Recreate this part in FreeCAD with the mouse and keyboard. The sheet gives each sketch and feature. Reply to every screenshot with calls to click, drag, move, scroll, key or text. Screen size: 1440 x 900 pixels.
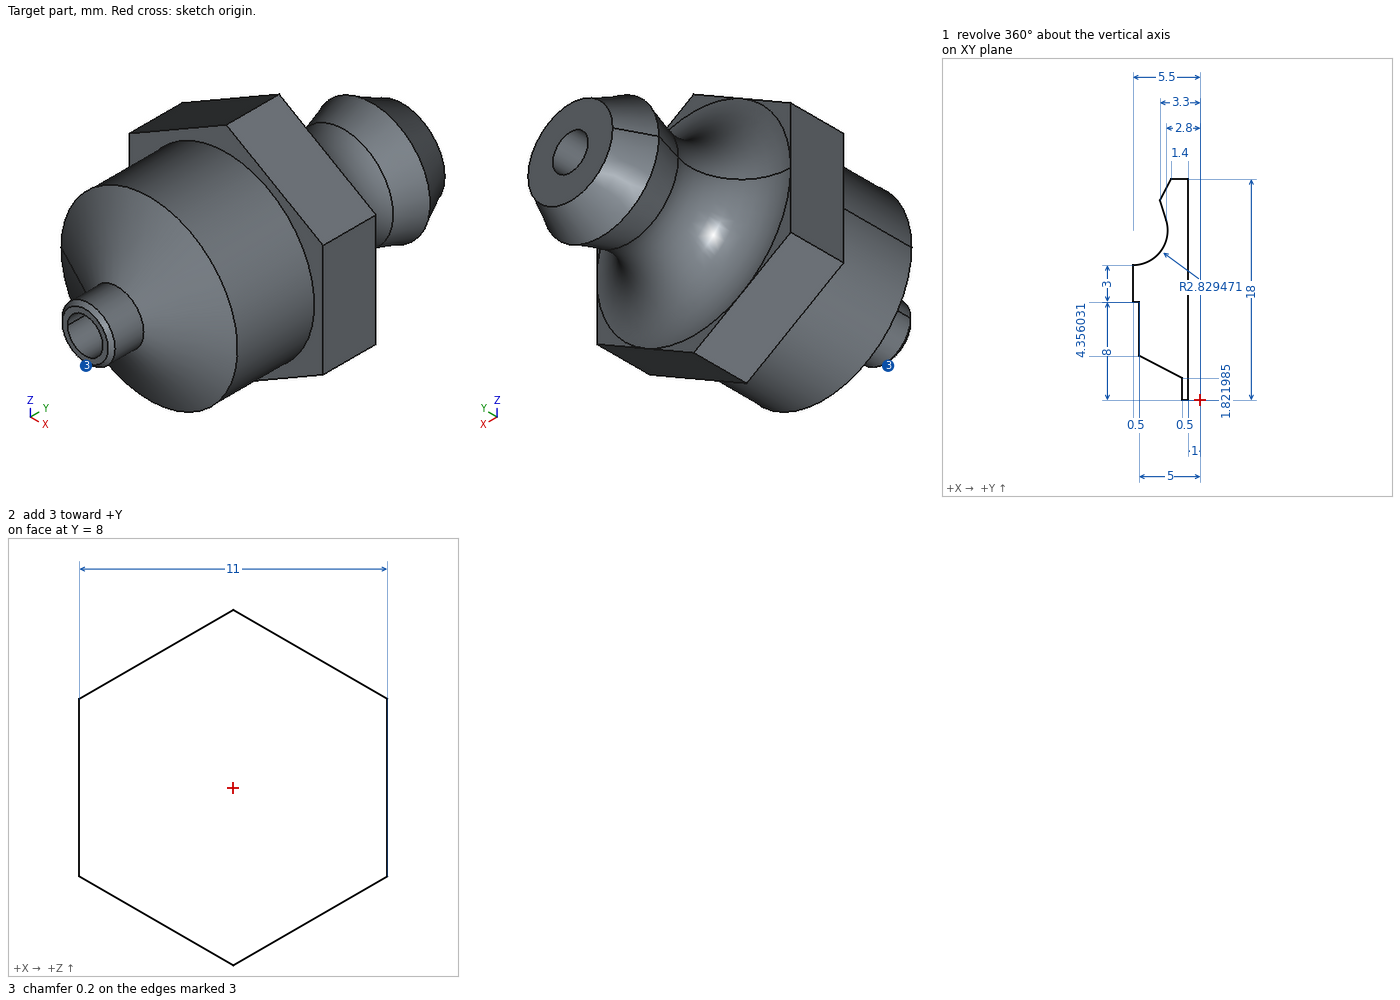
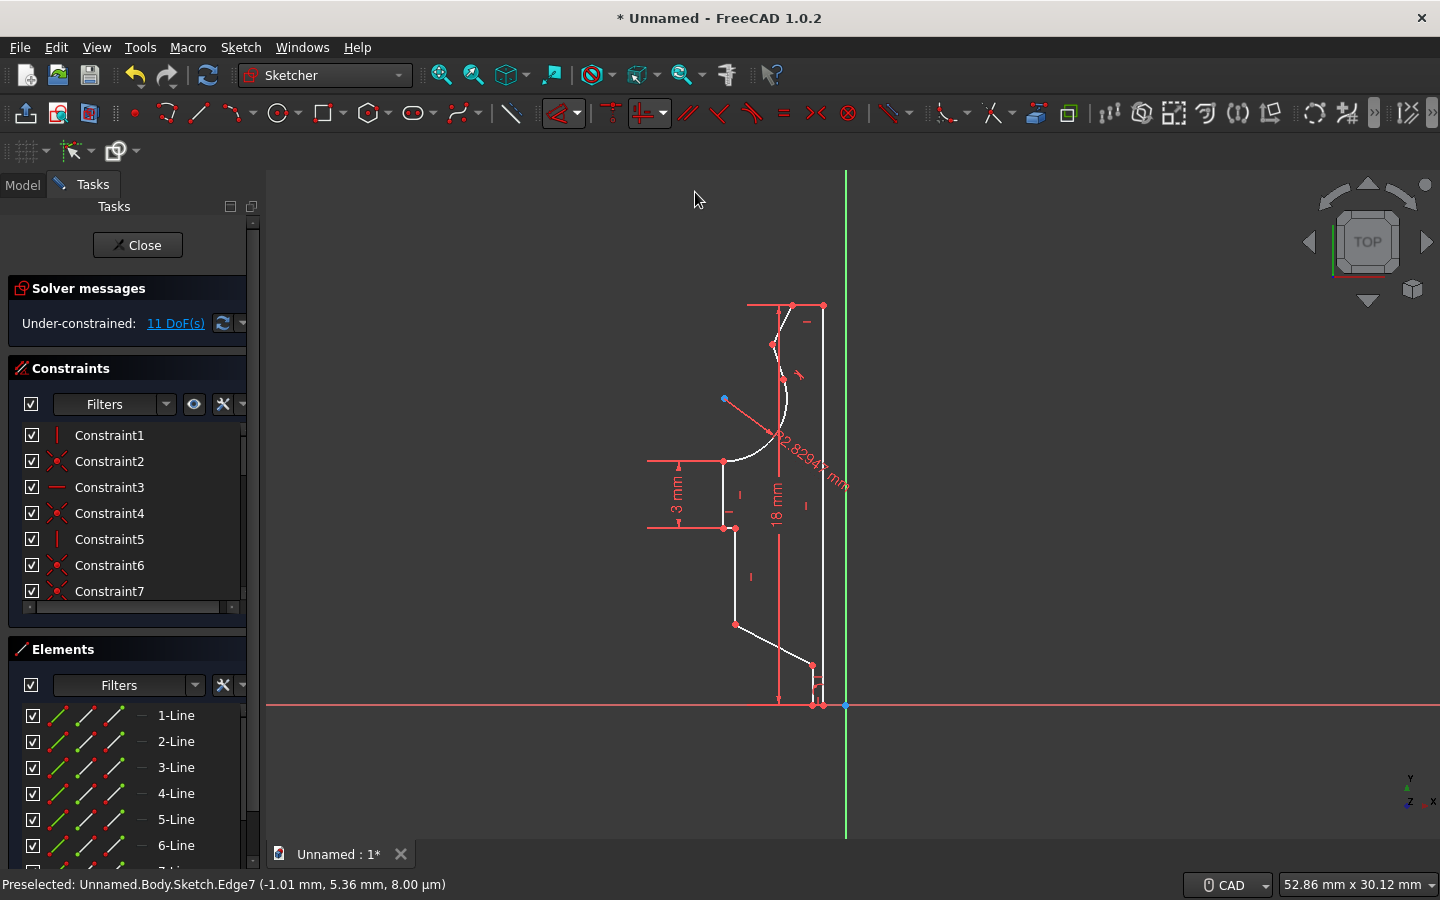
click(723, 528)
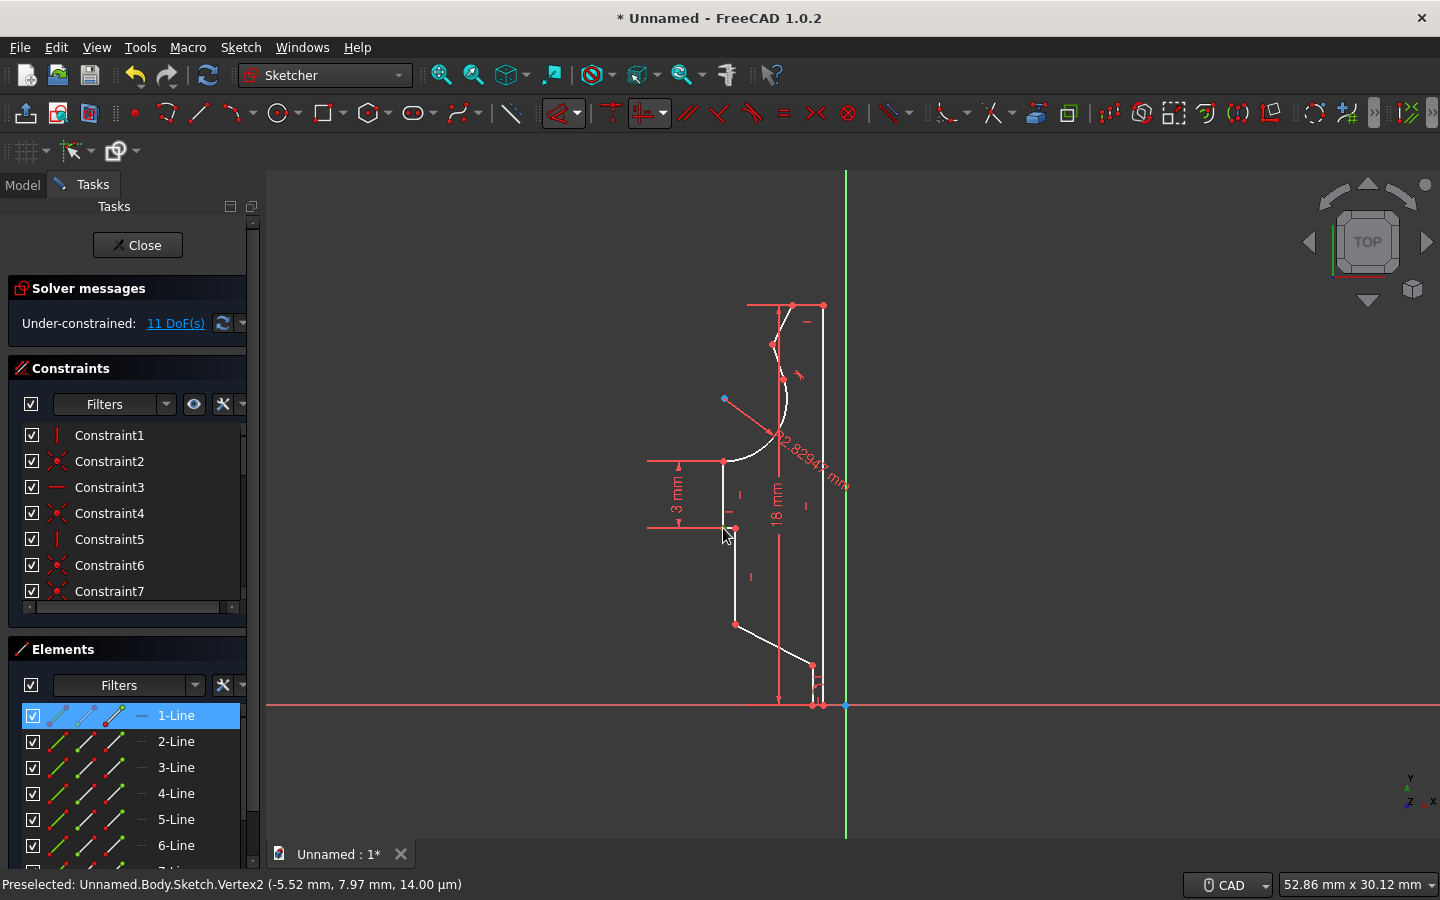
click(580, 114)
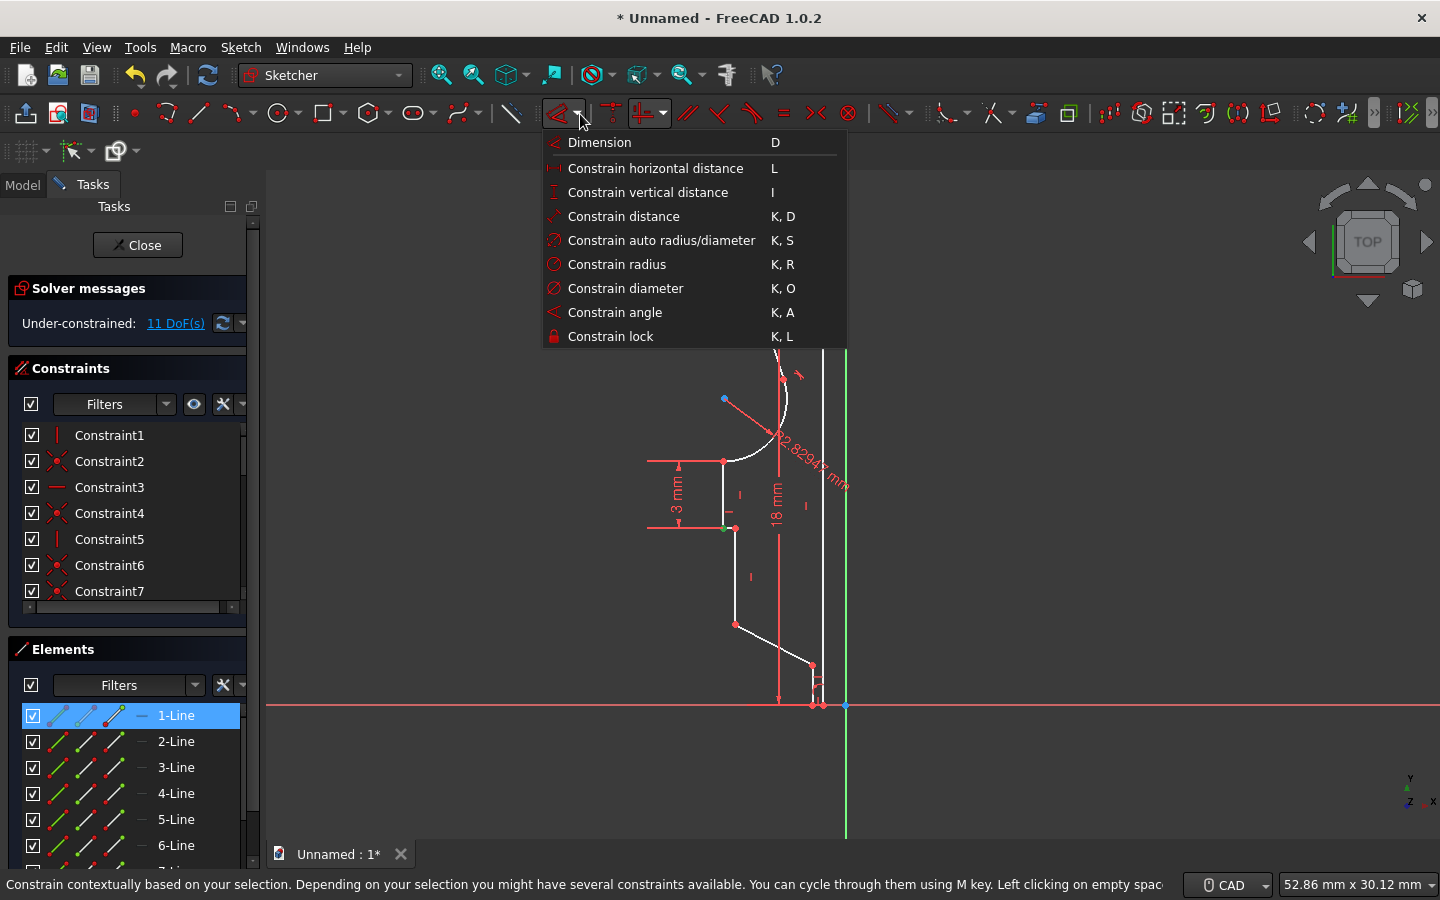
click(695, 192)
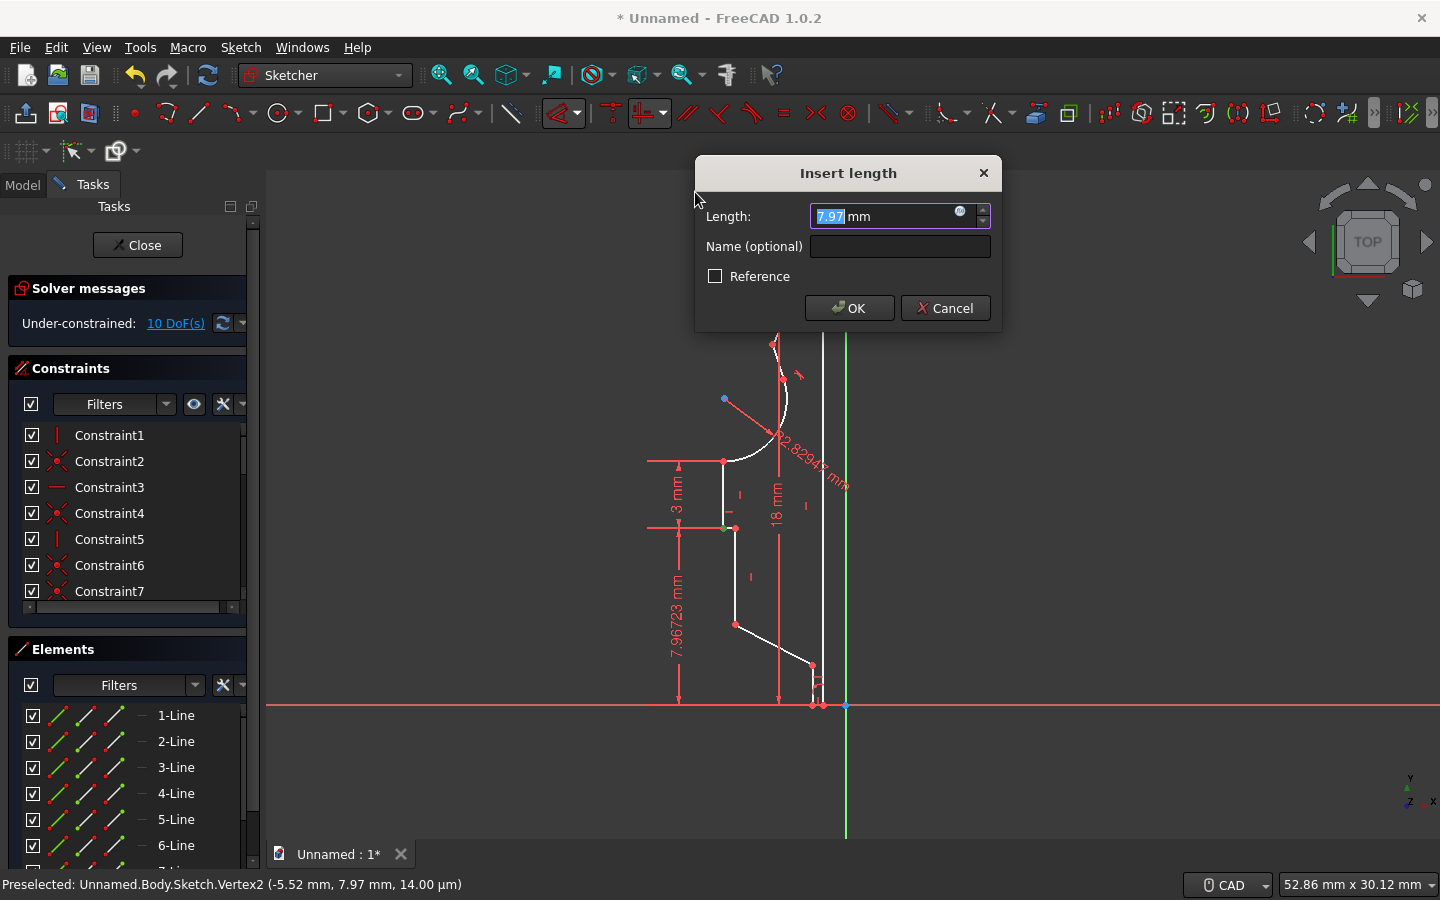
text(8)
key(Return)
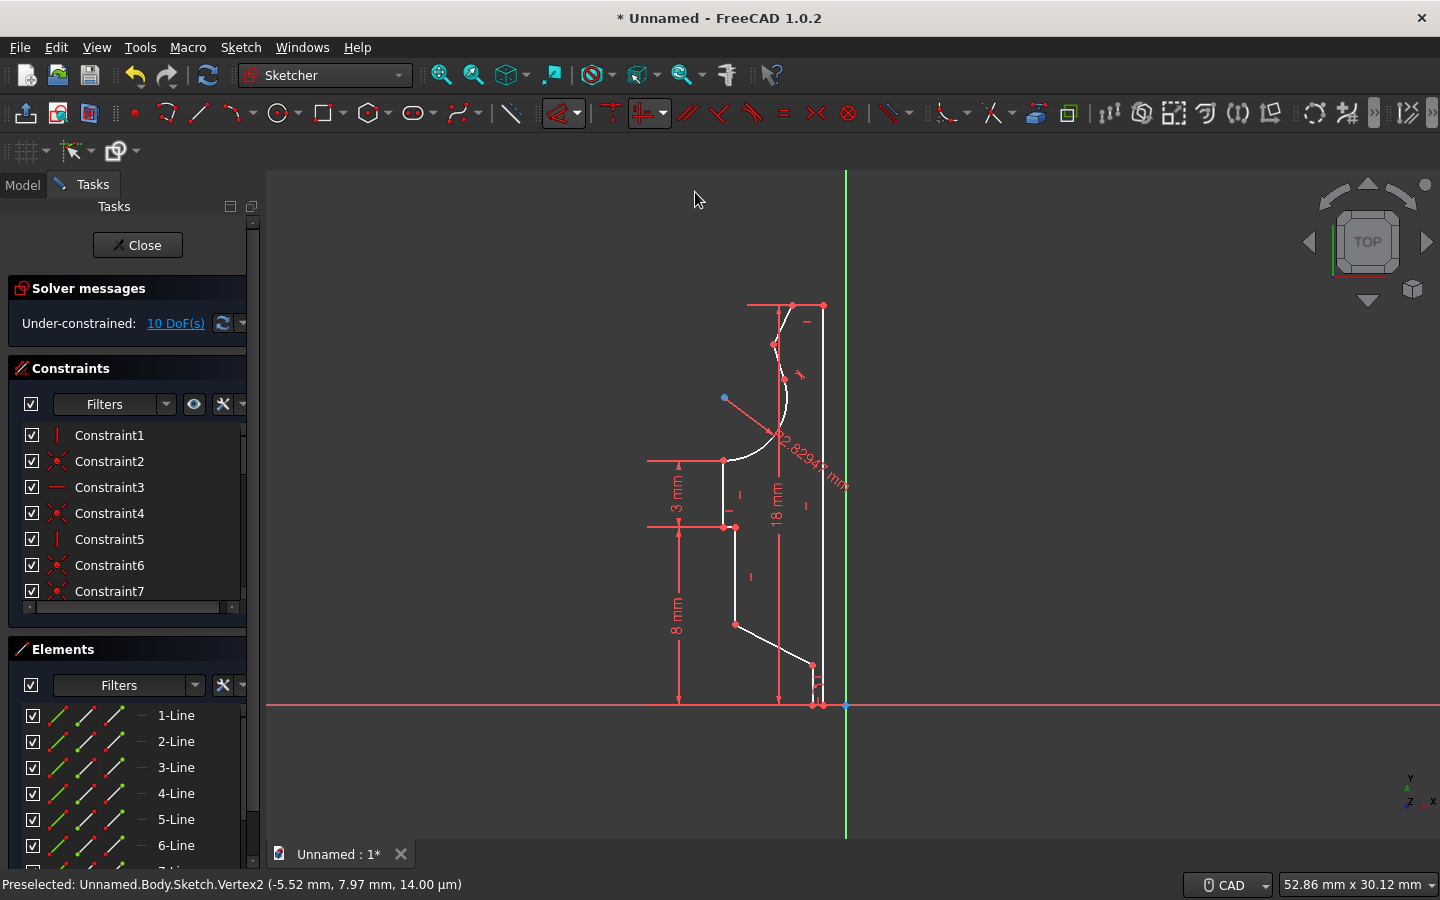
click(735, 527)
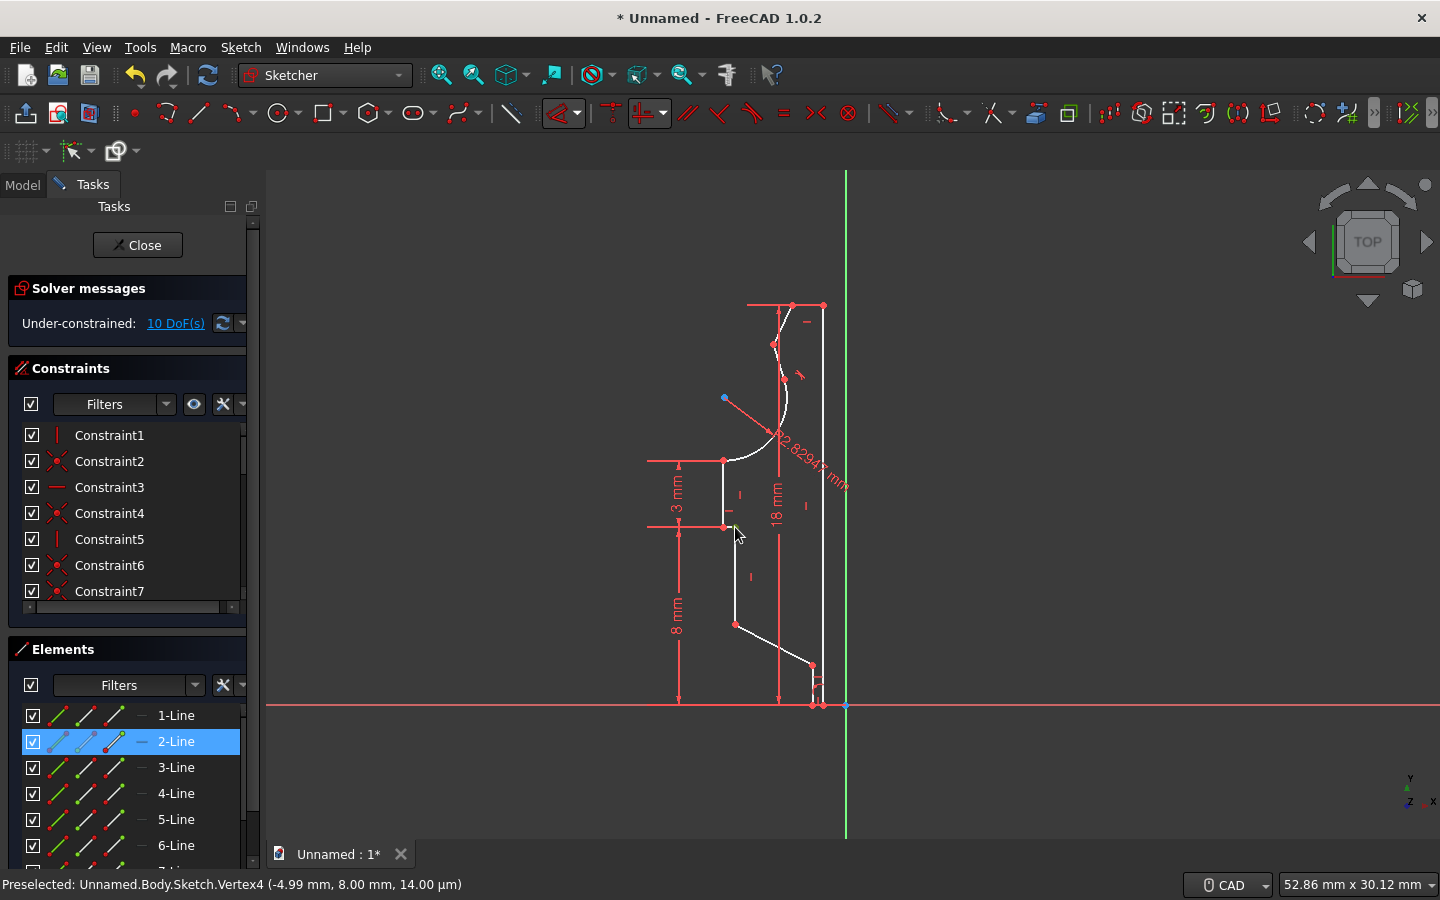
key(l)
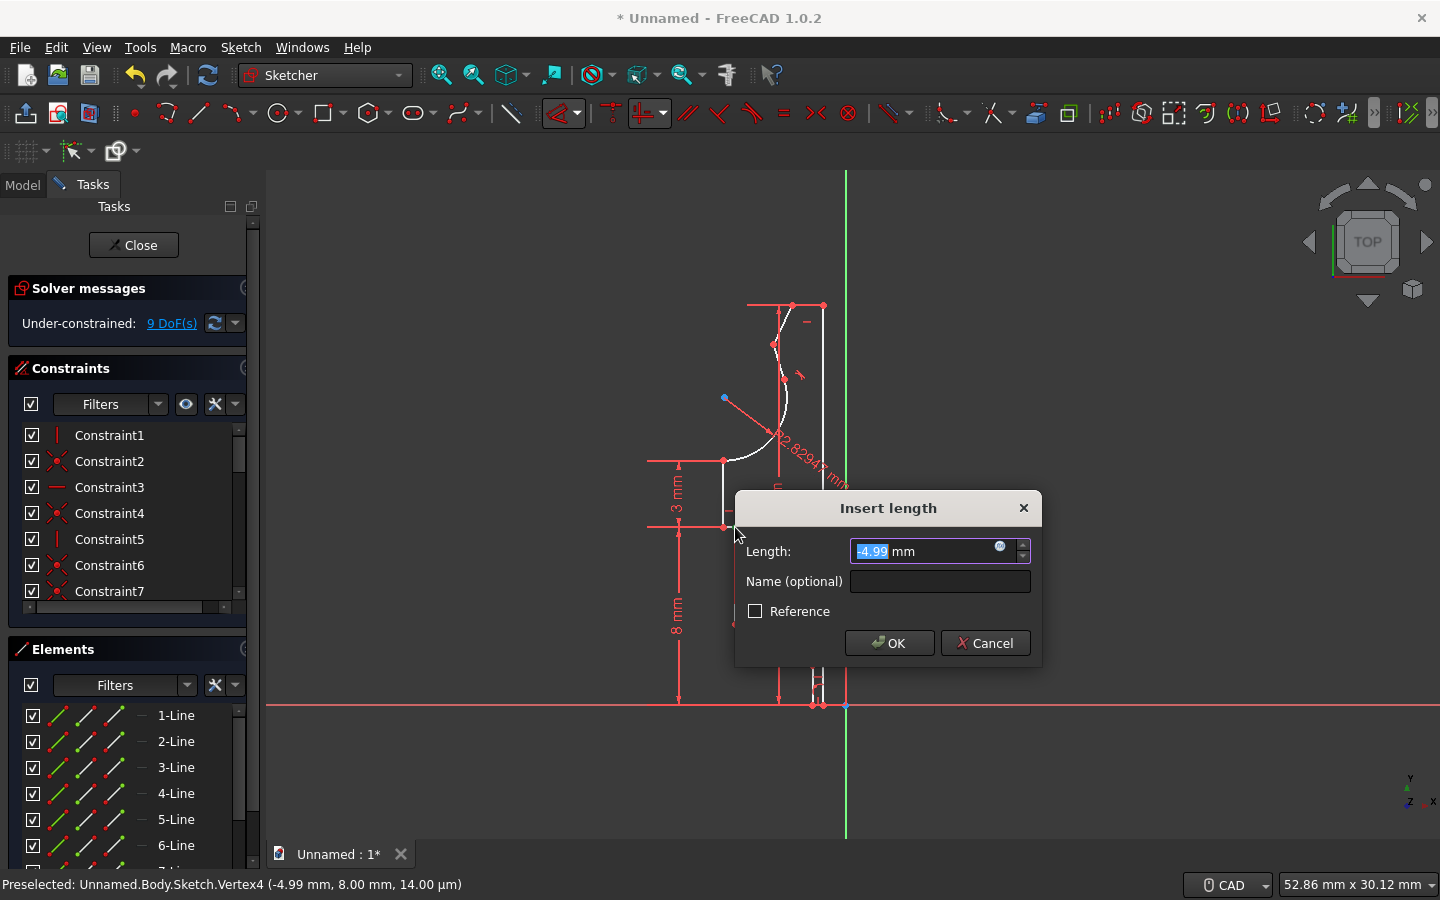
text(-5)
key(Return)